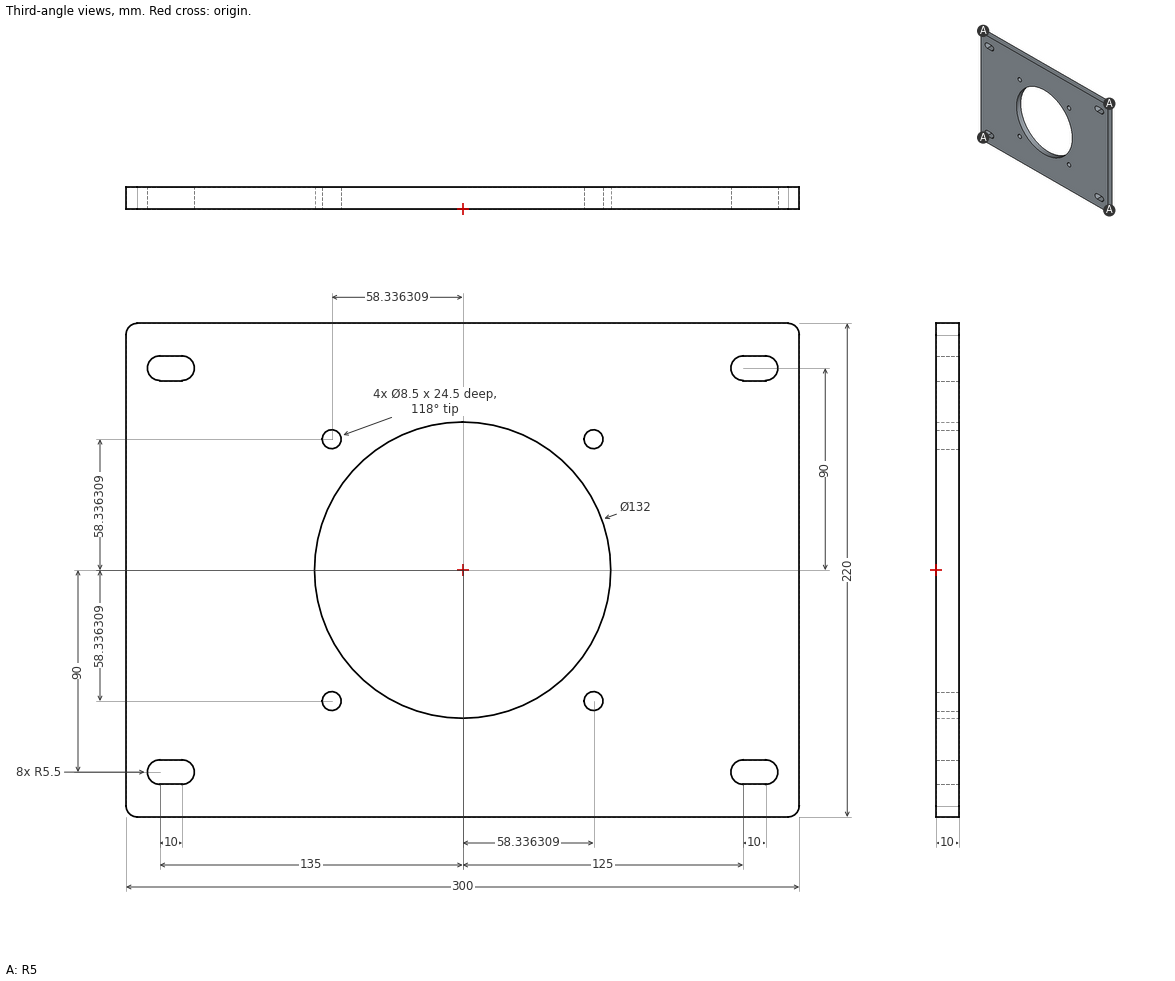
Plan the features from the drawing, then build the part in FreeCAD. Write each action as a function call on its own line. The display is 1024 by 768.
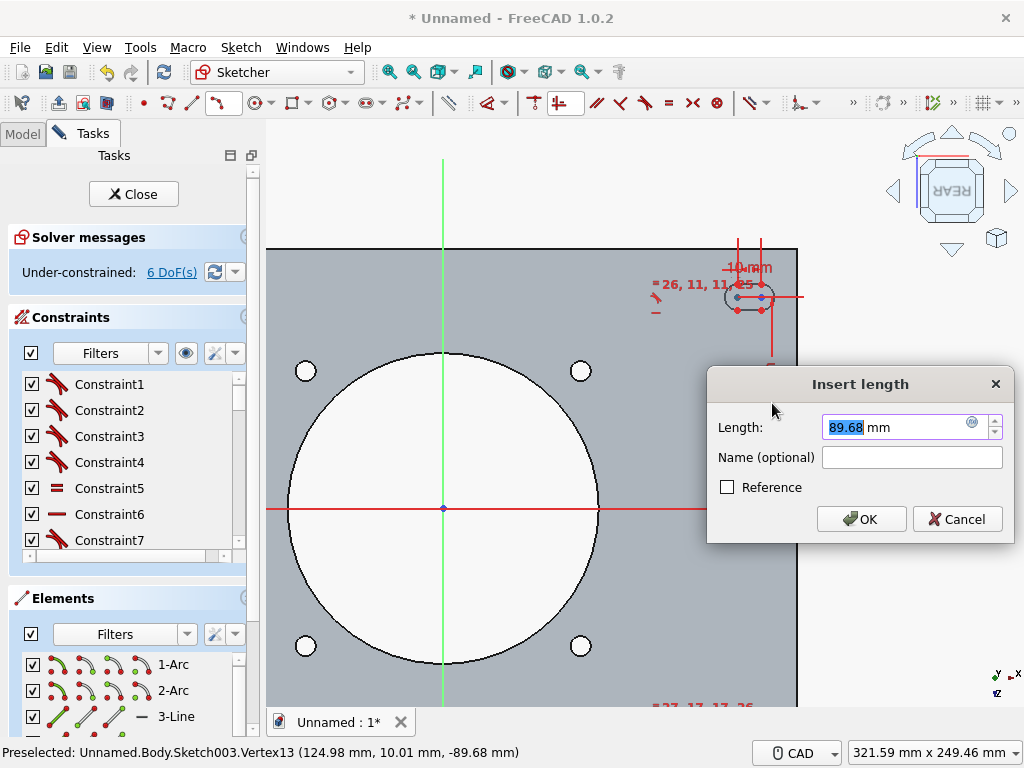
text(90)
key(Return)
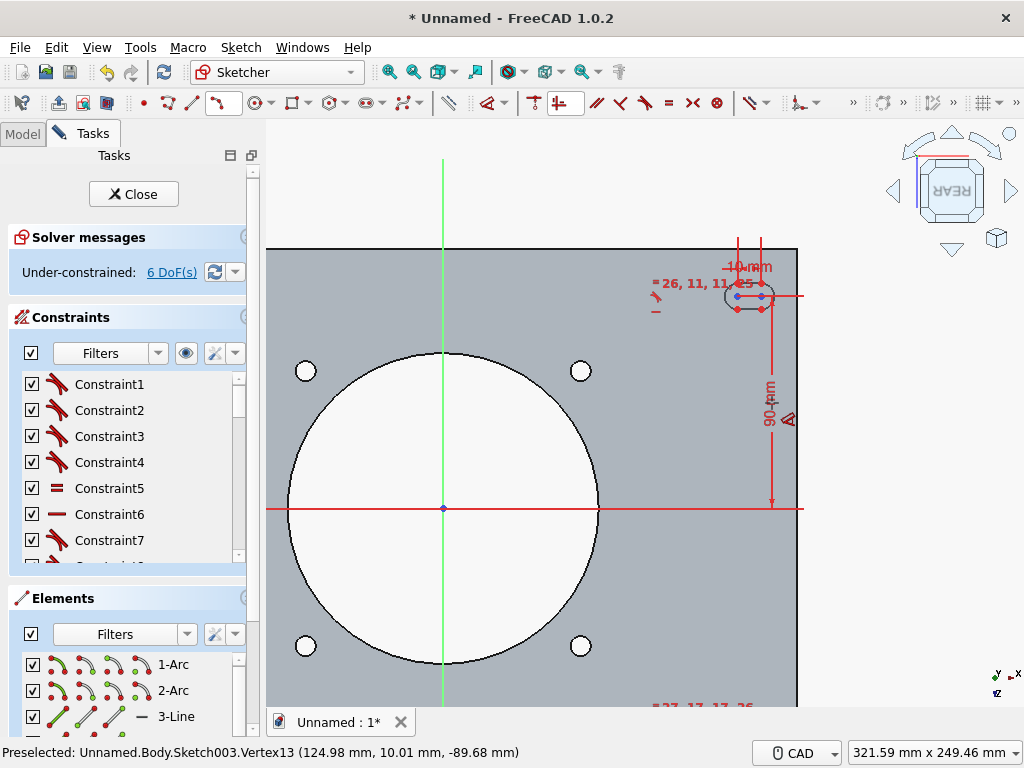
scroll(739, 297, down, 3)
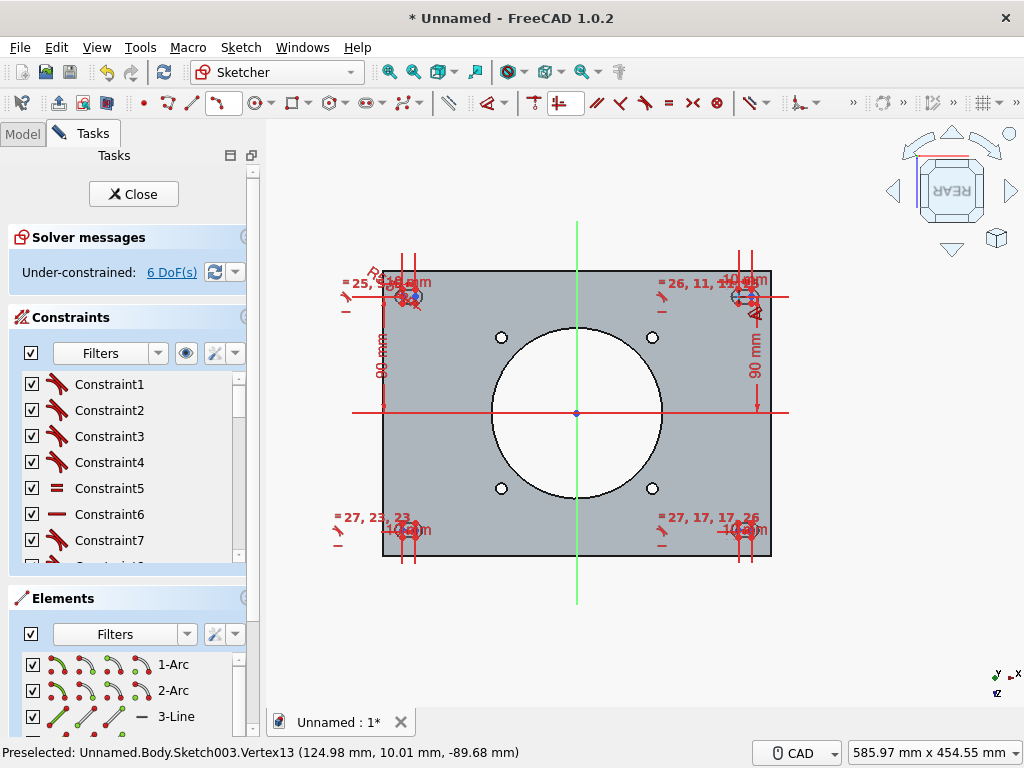
scroll(739, 530, up, 3)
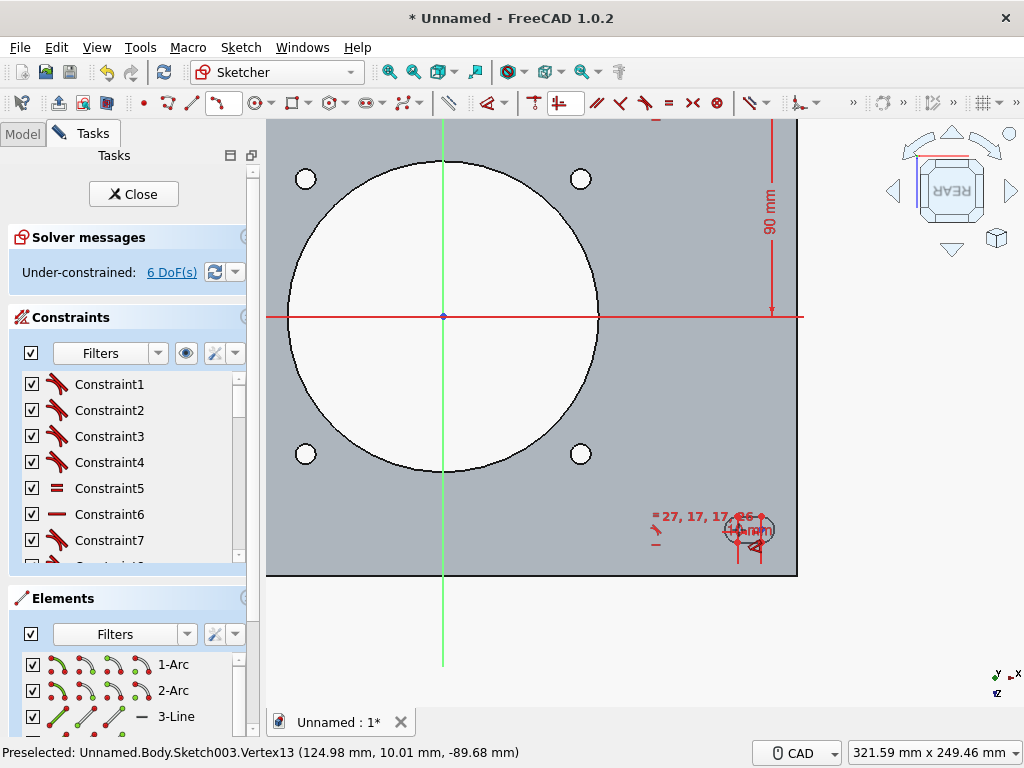
click(738, 530)
click(772, 423)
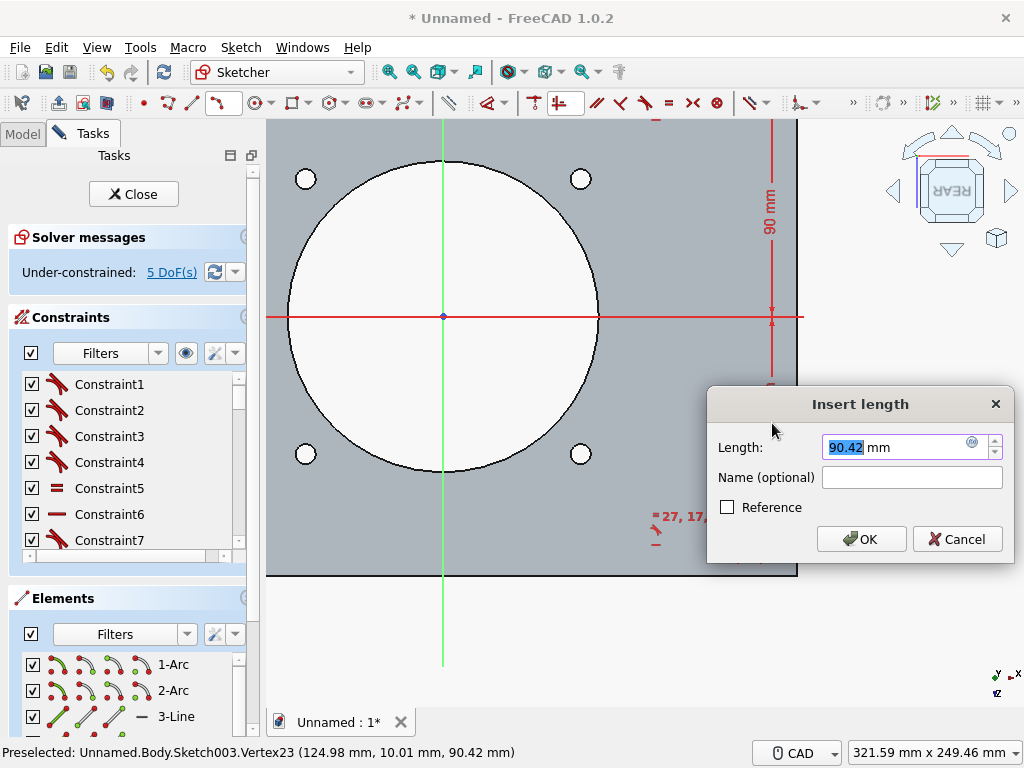
text(90)
key(Return)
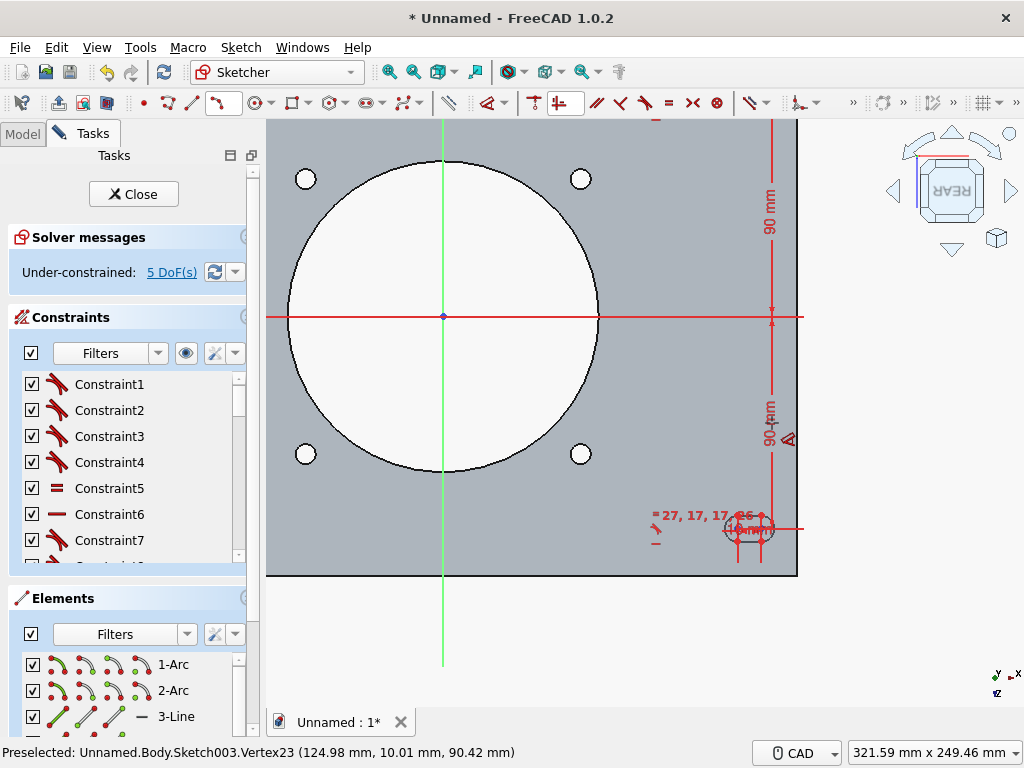
scroll(739, 530, down, 3)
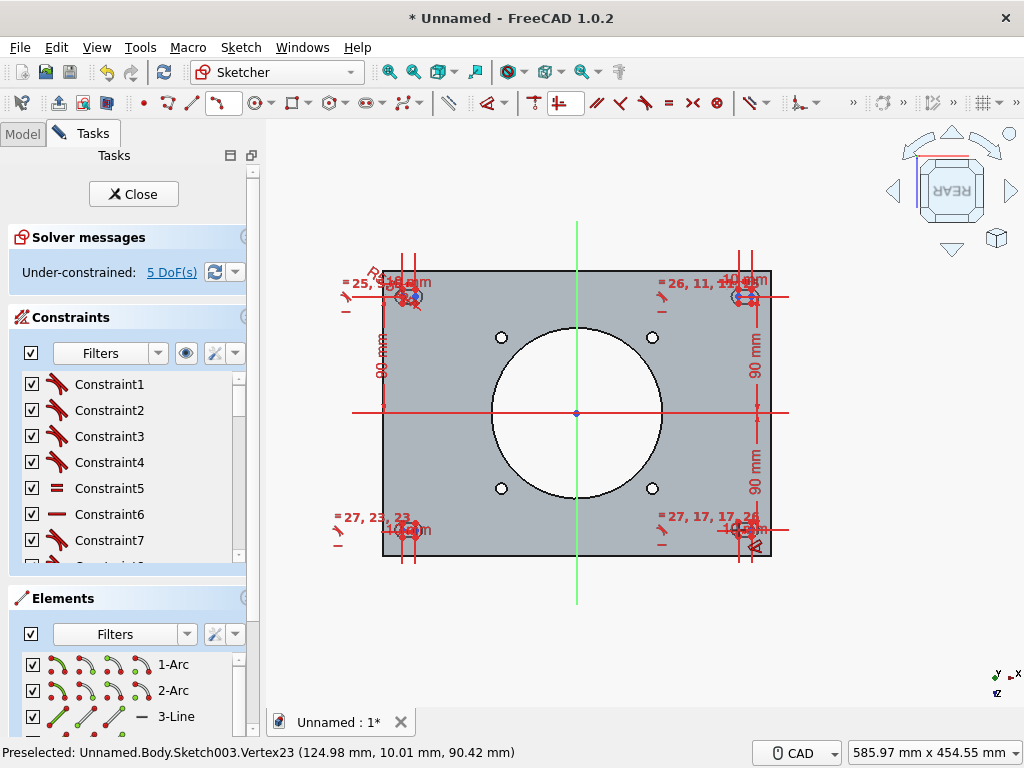
scroll(402, 530, up, 3)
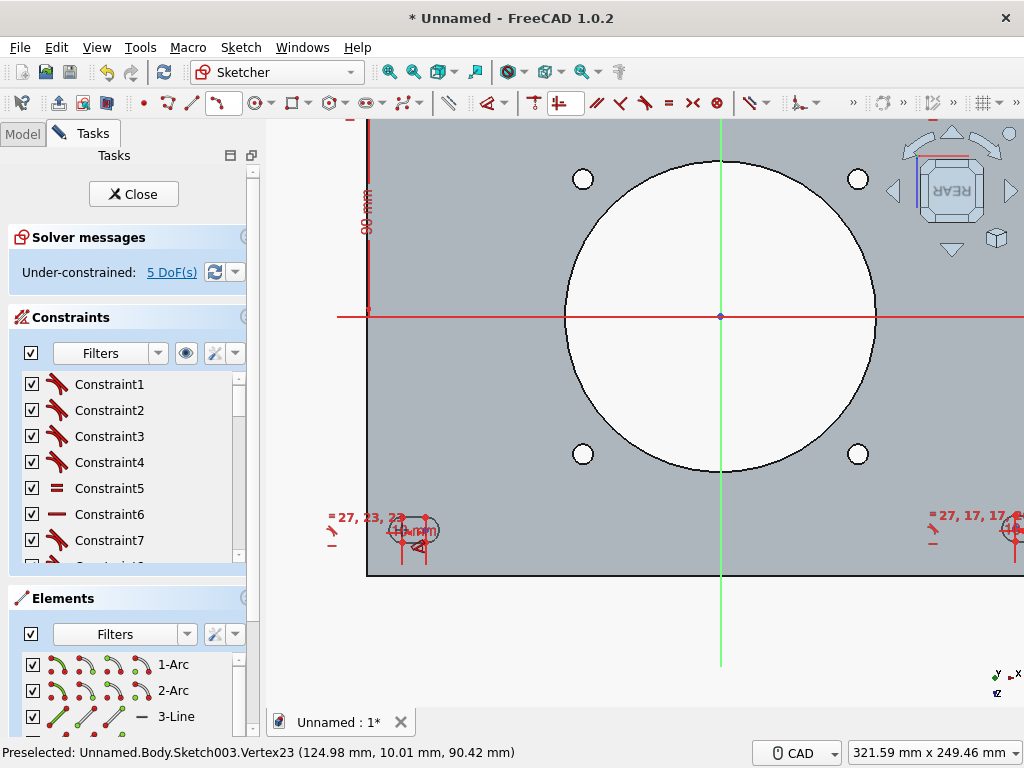
click(402, 530)
click(368, 423)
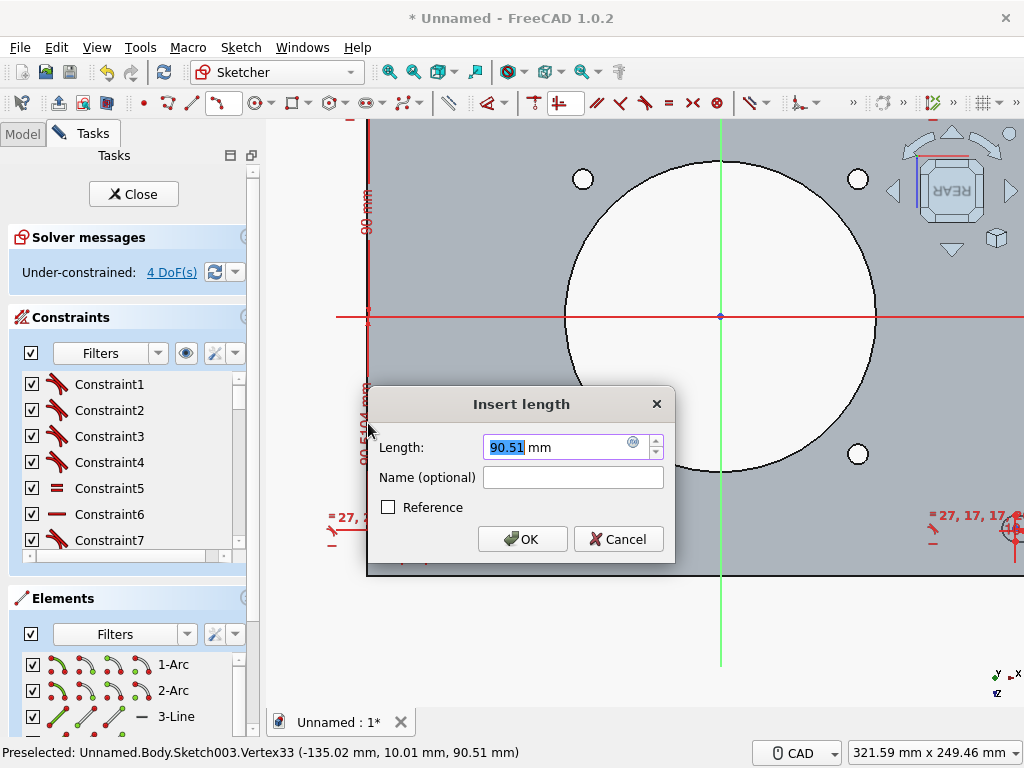
text(90)
key(Return)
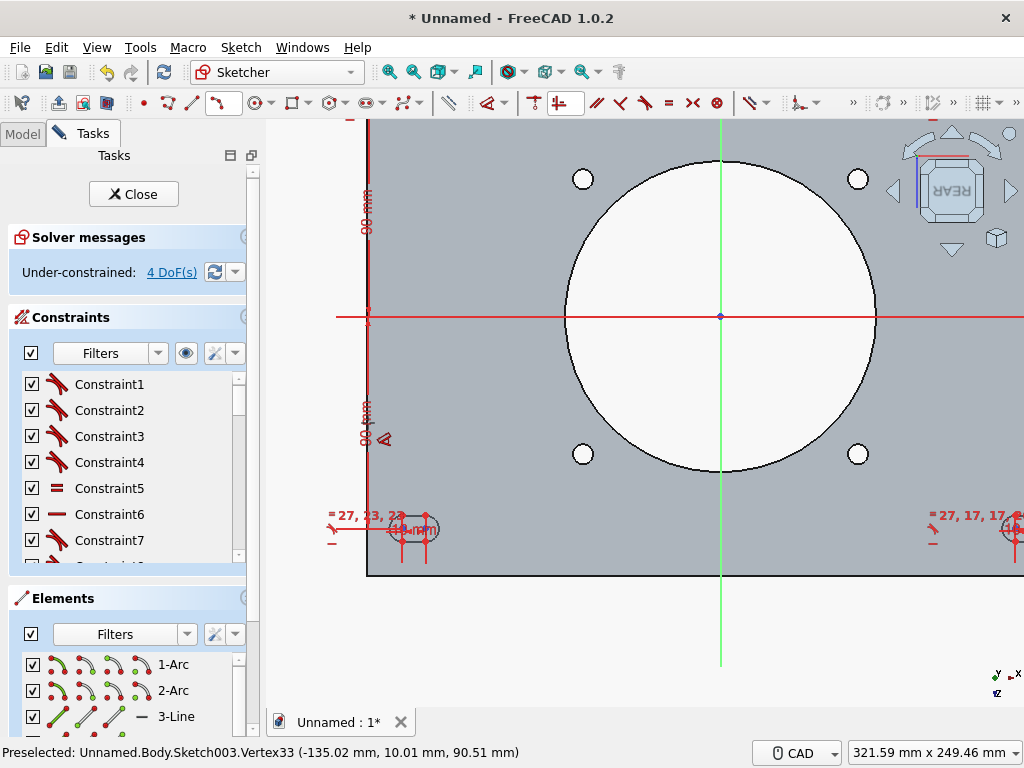
scroll(401, 530, down, 3)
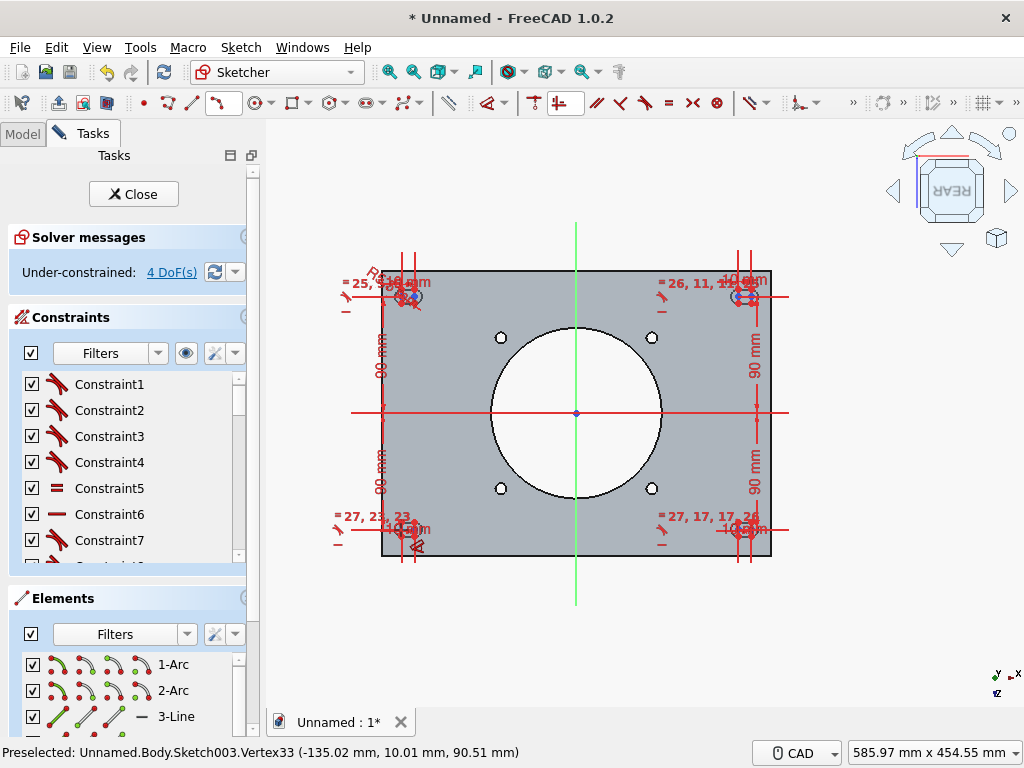
scroll(402, 290, up, 3)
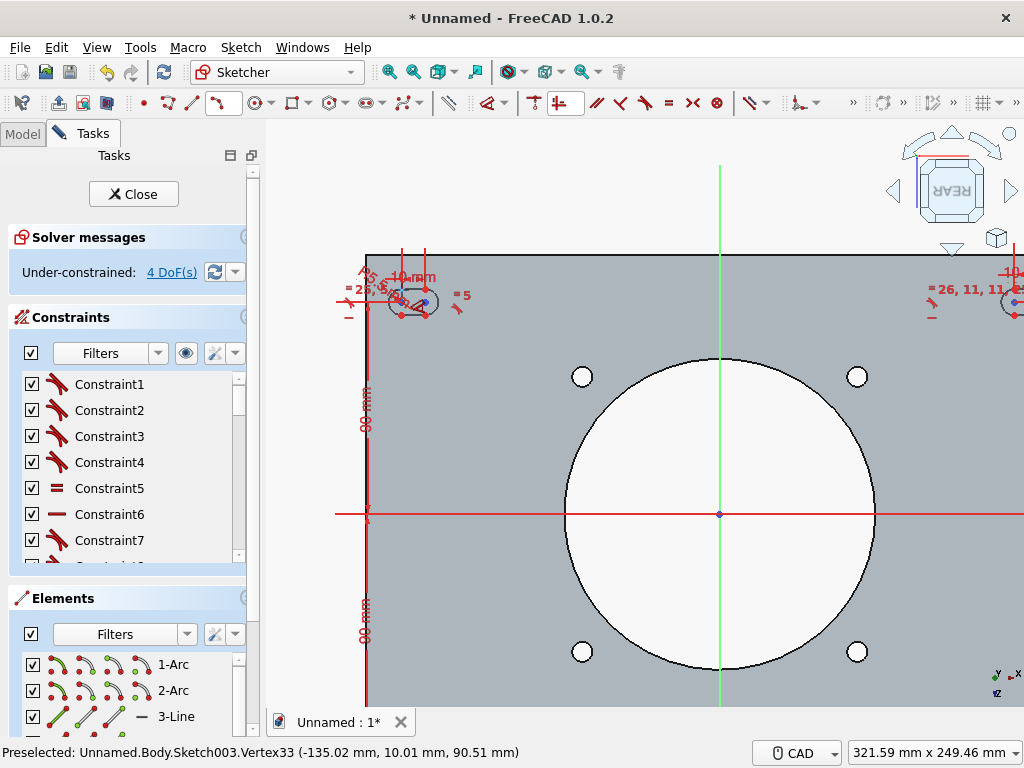
click(402, 289)
click(561, 255)